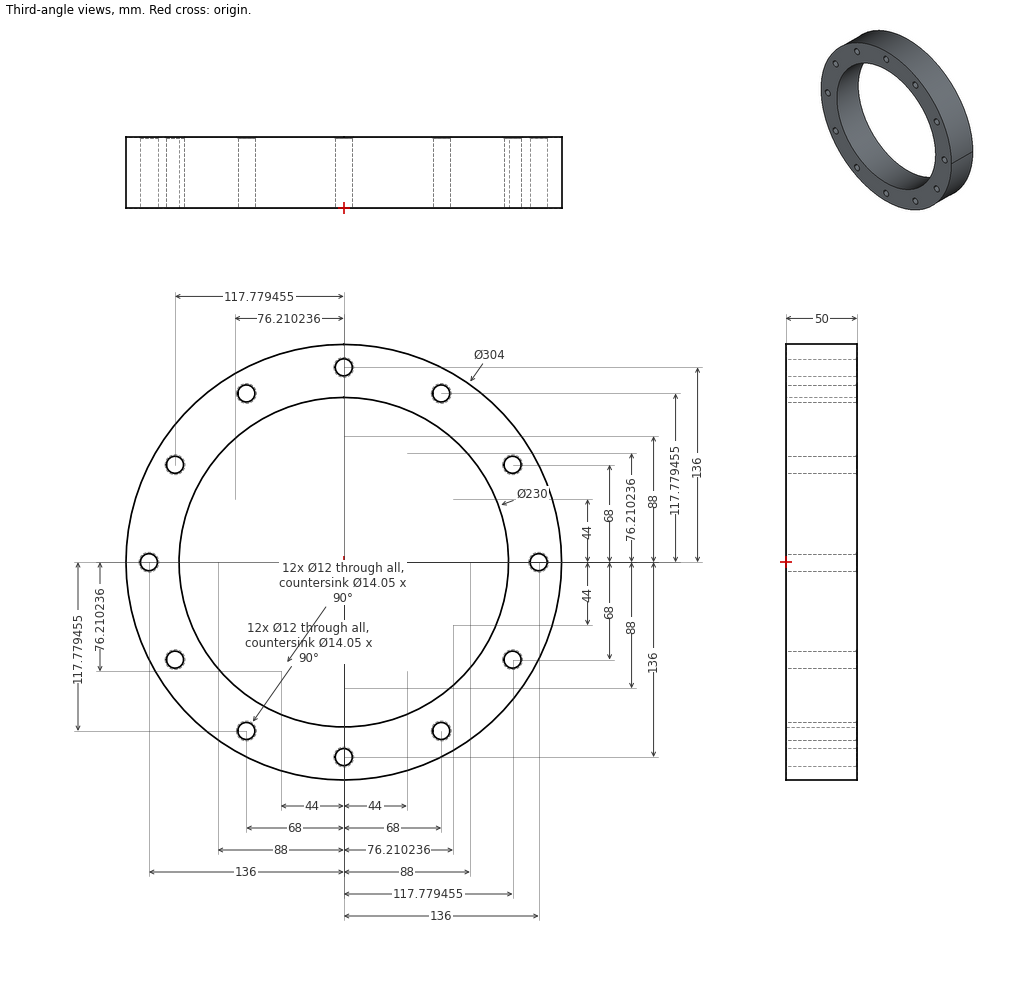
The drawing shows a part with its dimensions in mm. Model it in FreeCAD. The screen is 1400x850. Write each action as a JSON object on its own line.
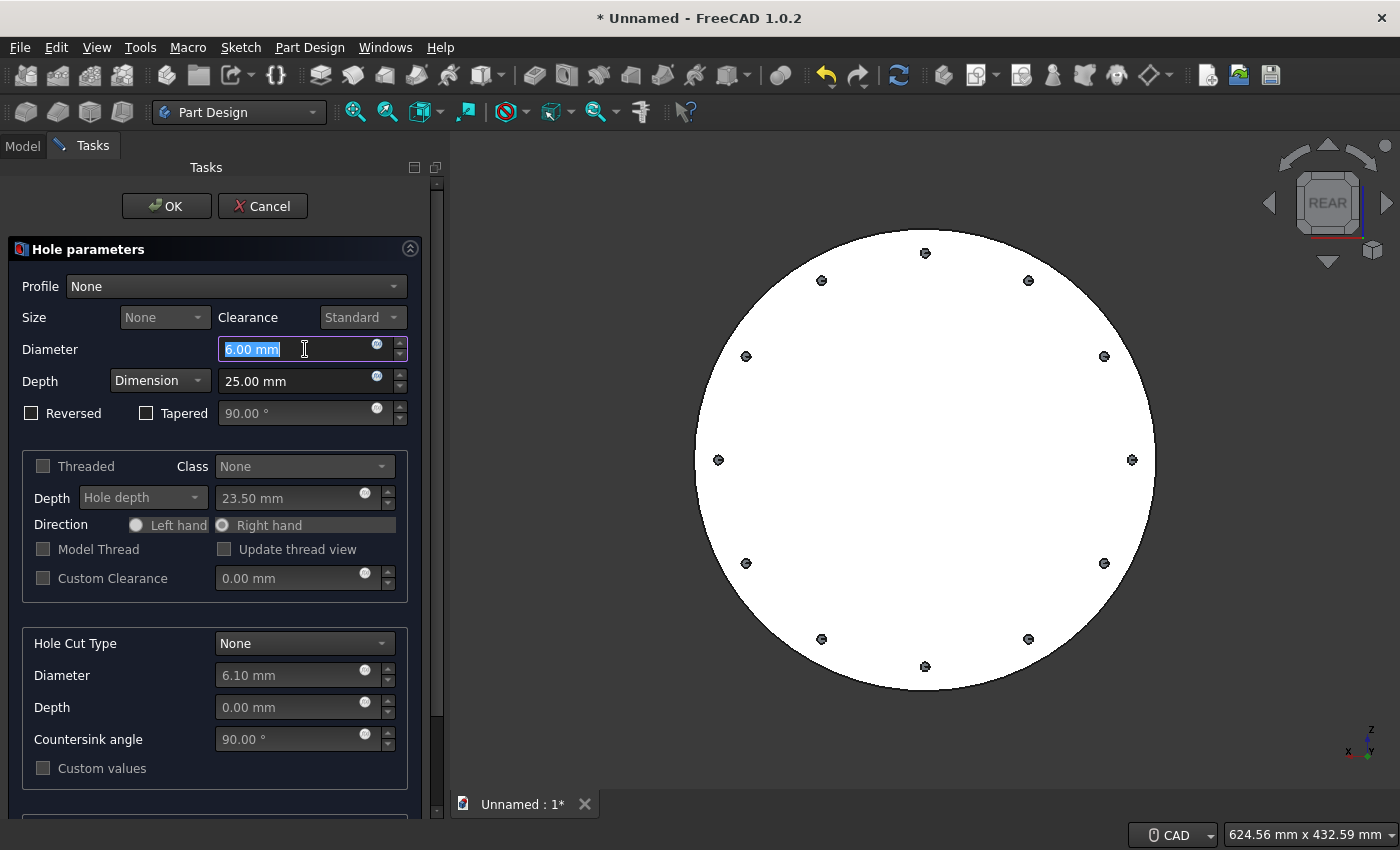
{"action": "type", "text": "12"}
{"action": "key", "text": "Tab"}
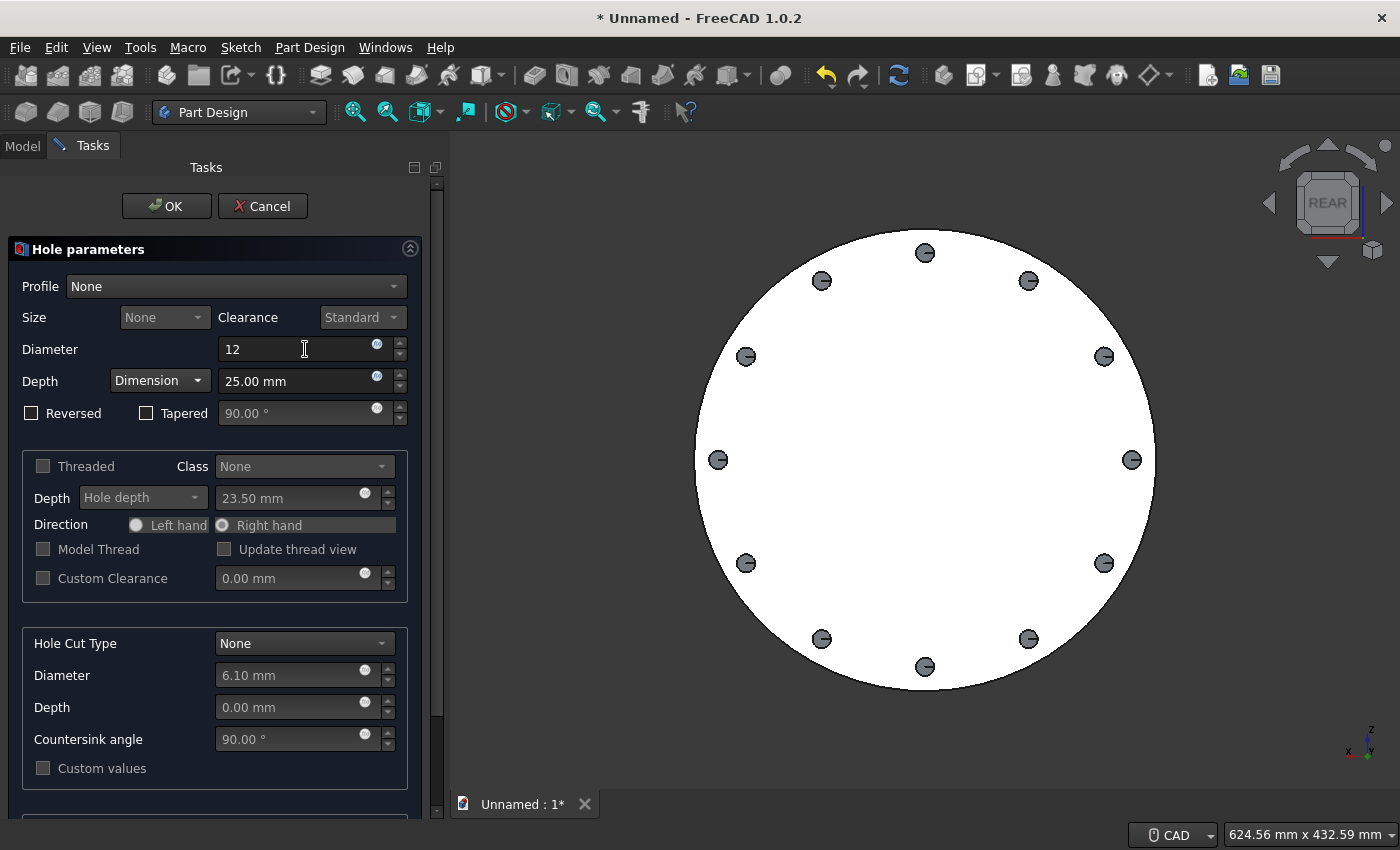
{"action": "left_click", "coordinate": [161, 380]}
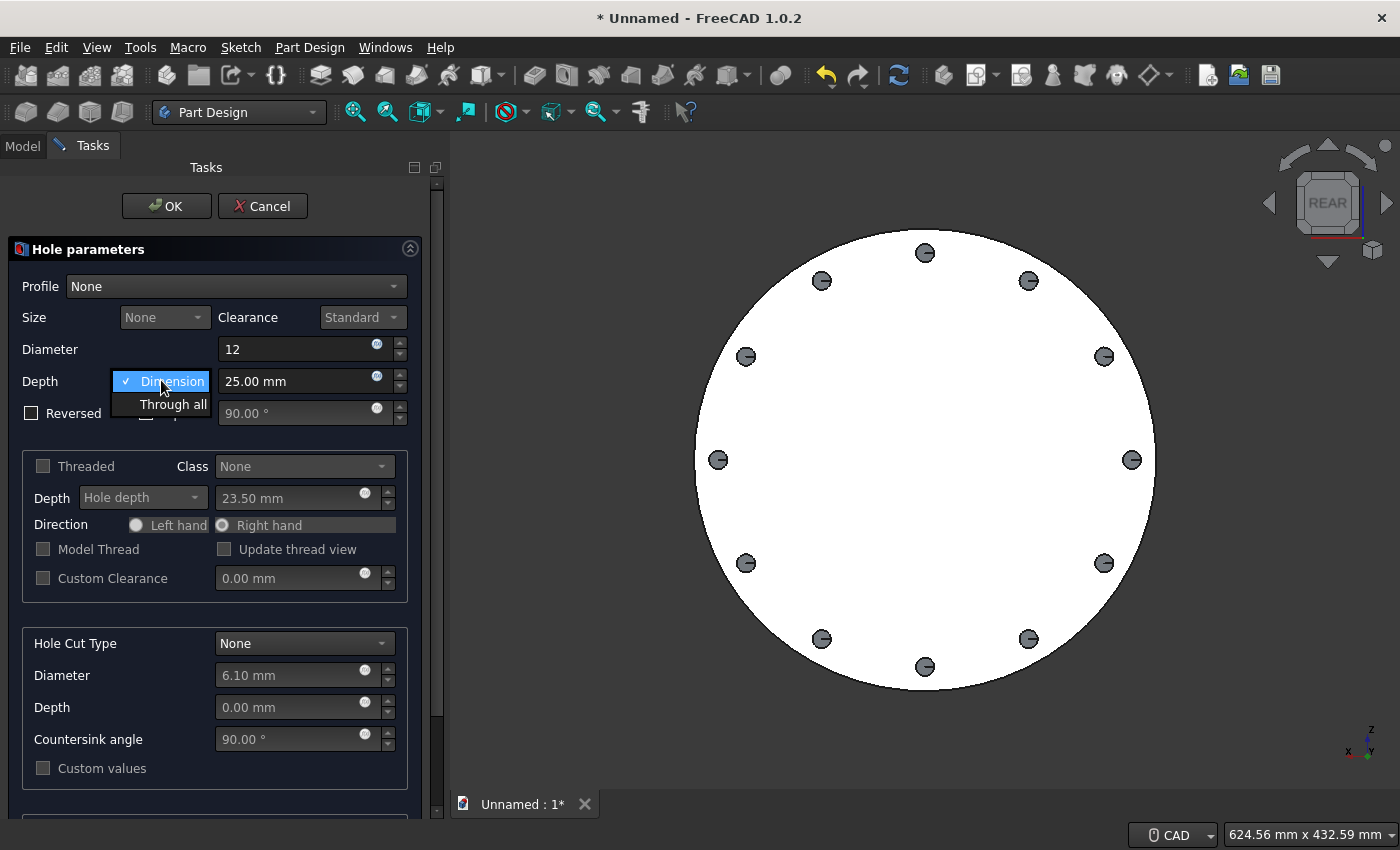
{"action": "left_click", "coordinate": [160, 404]}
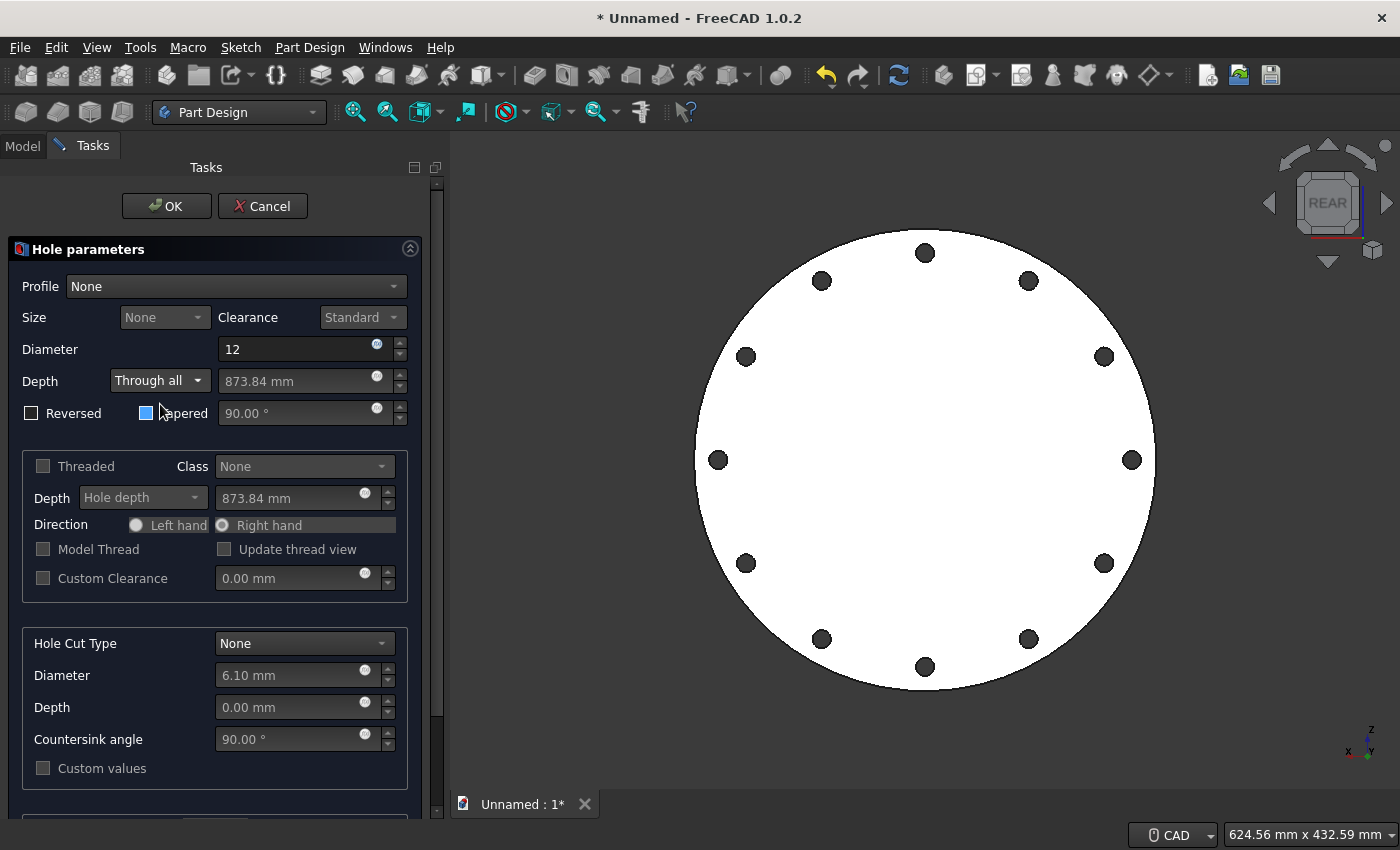
{"action": "left_click", "coordinate": [306, 644]}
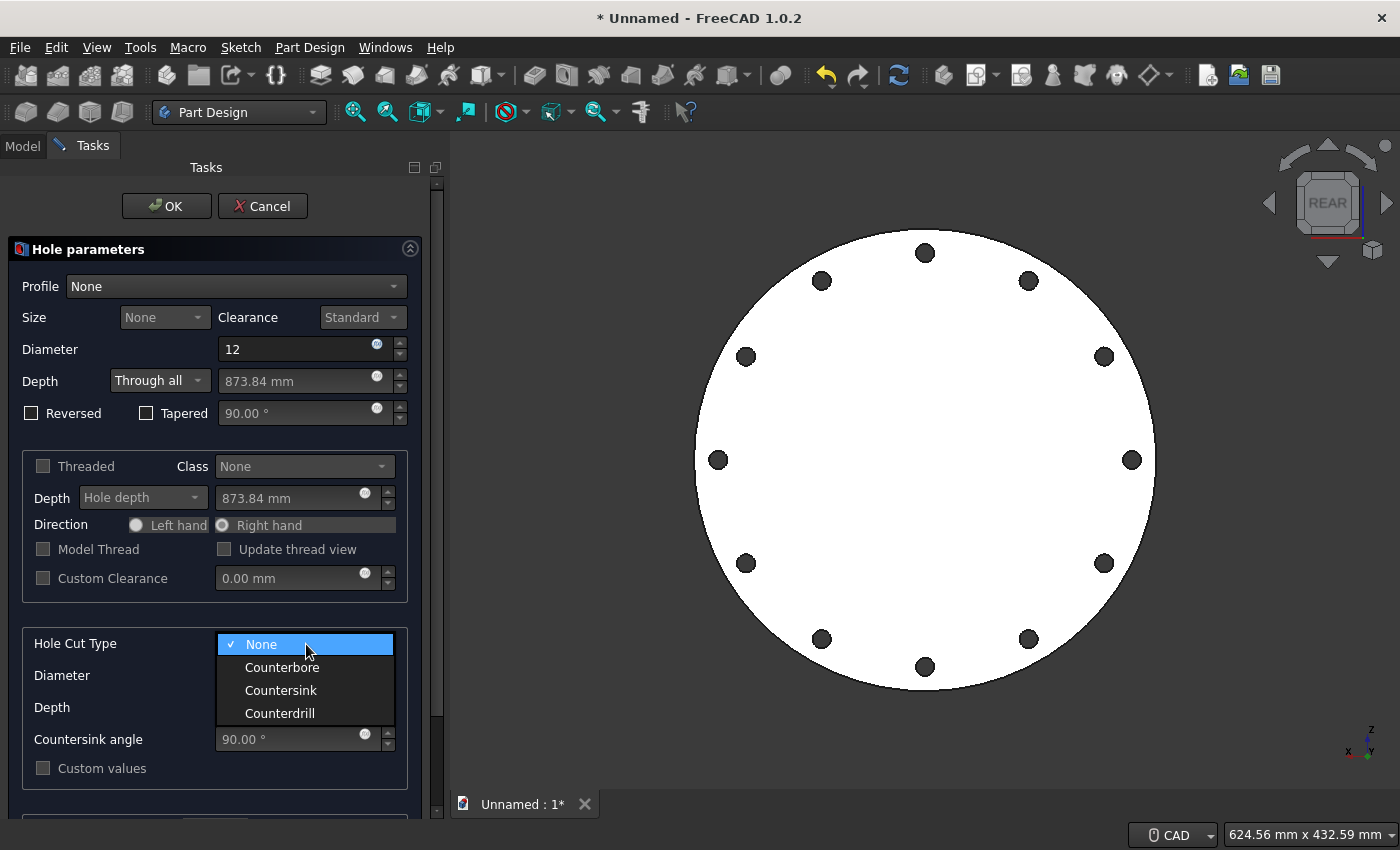
{"action": "left_click", "coordinate": [304, 690]}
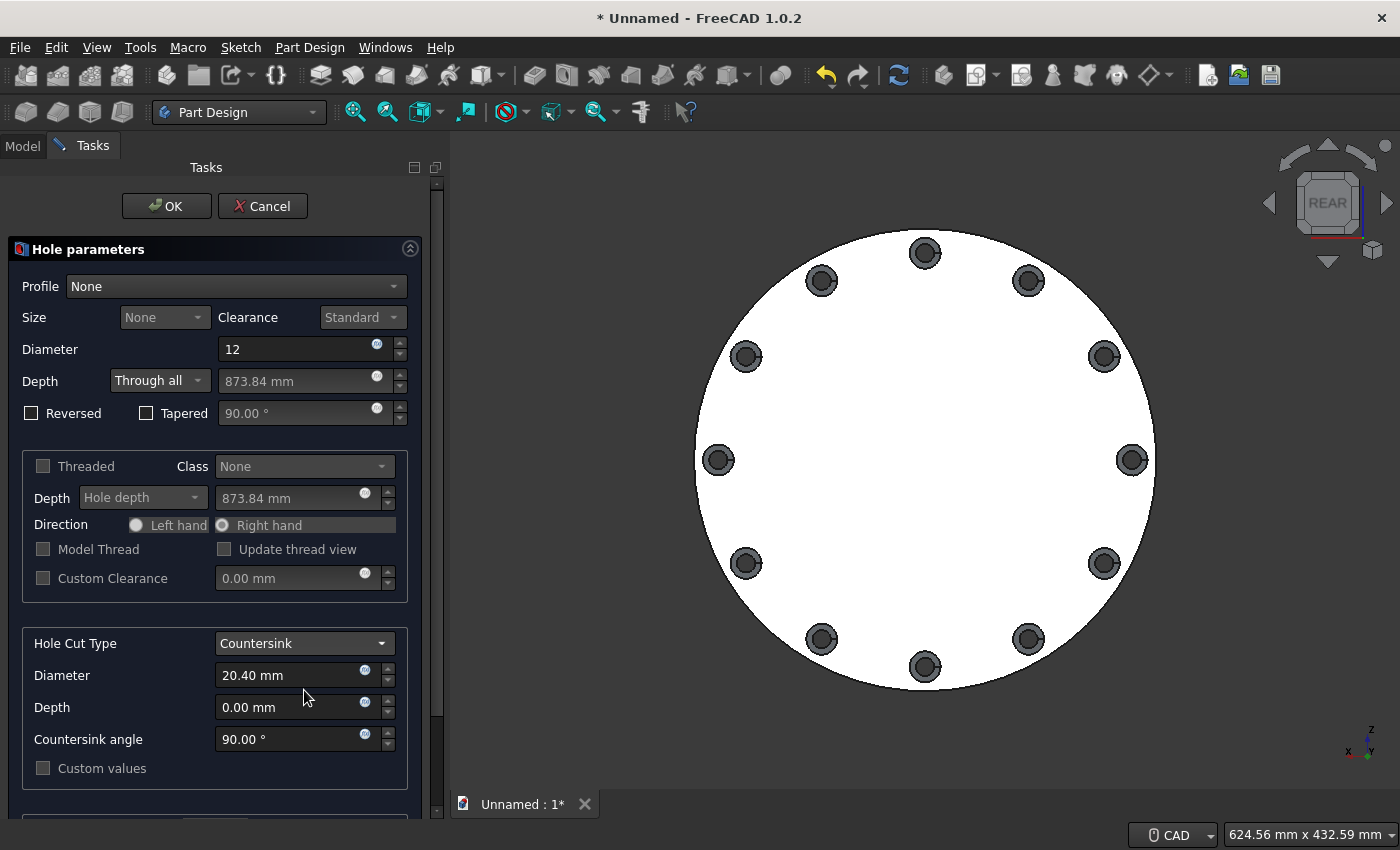
{"action": "triple_click", "coordinate": [298, 675]}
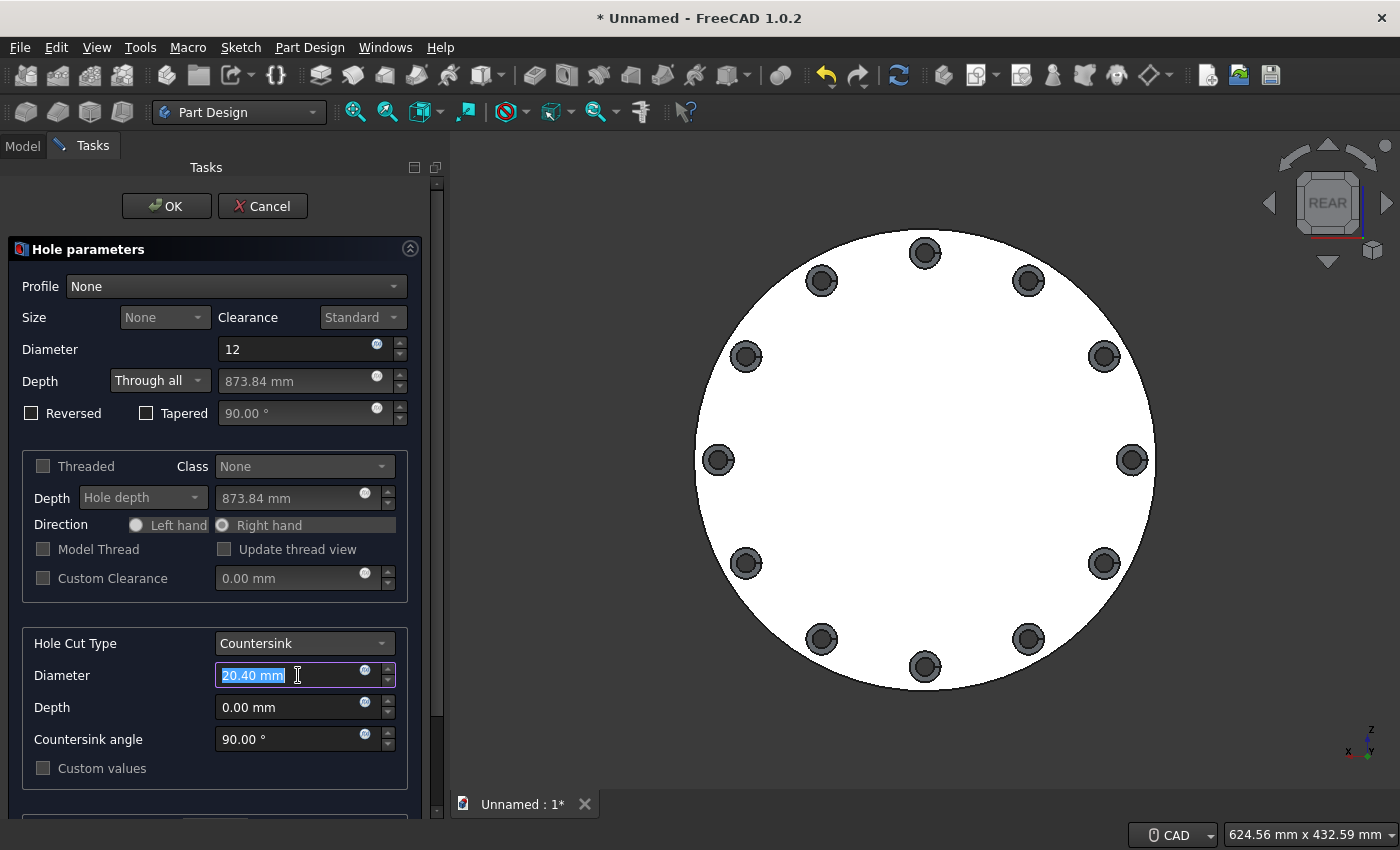
{"action": "type", "text": "14.05"}
{"action": "key", "text": "Tab"}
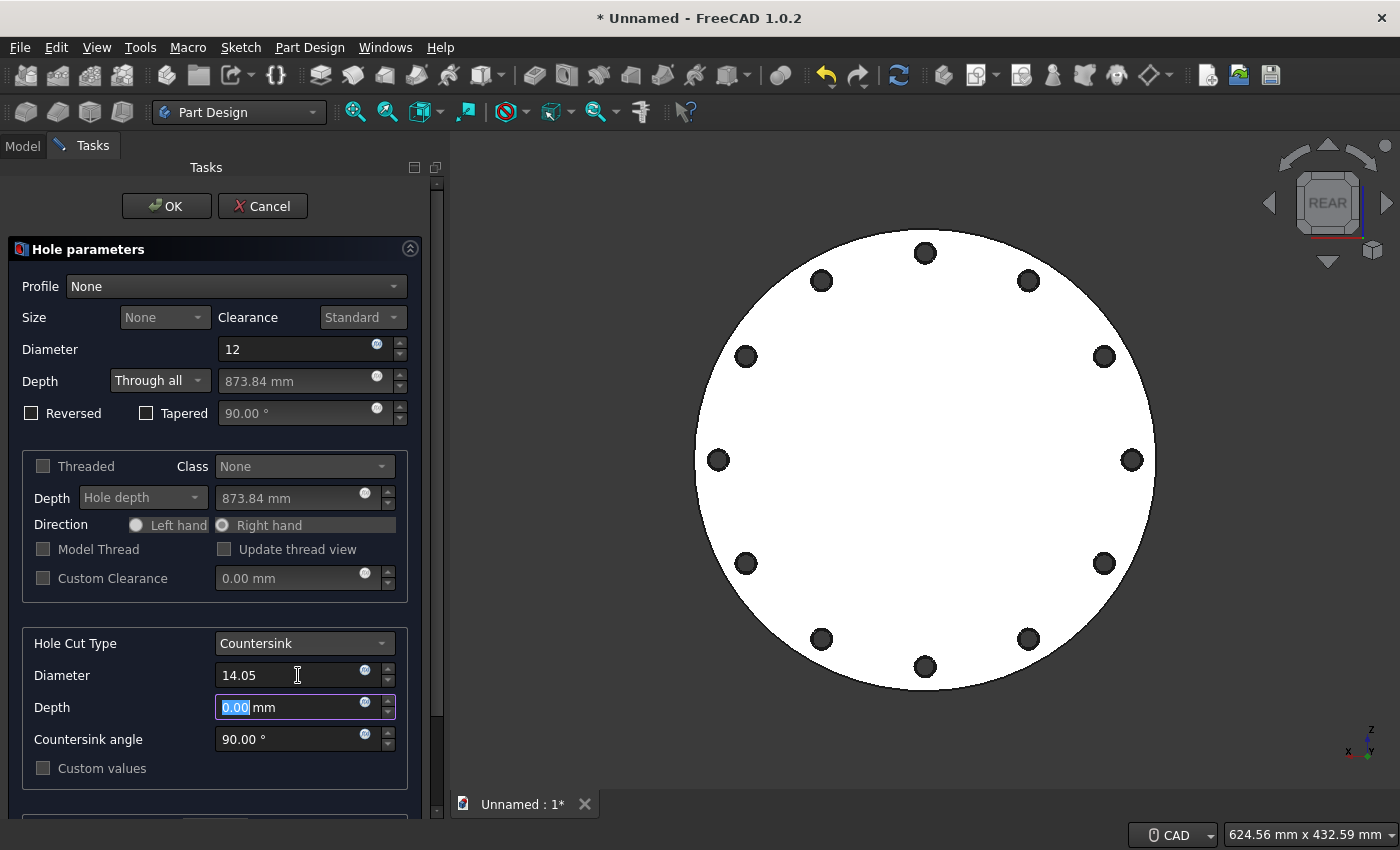
{"action": "left_click", "coordinate": [167, 206]}